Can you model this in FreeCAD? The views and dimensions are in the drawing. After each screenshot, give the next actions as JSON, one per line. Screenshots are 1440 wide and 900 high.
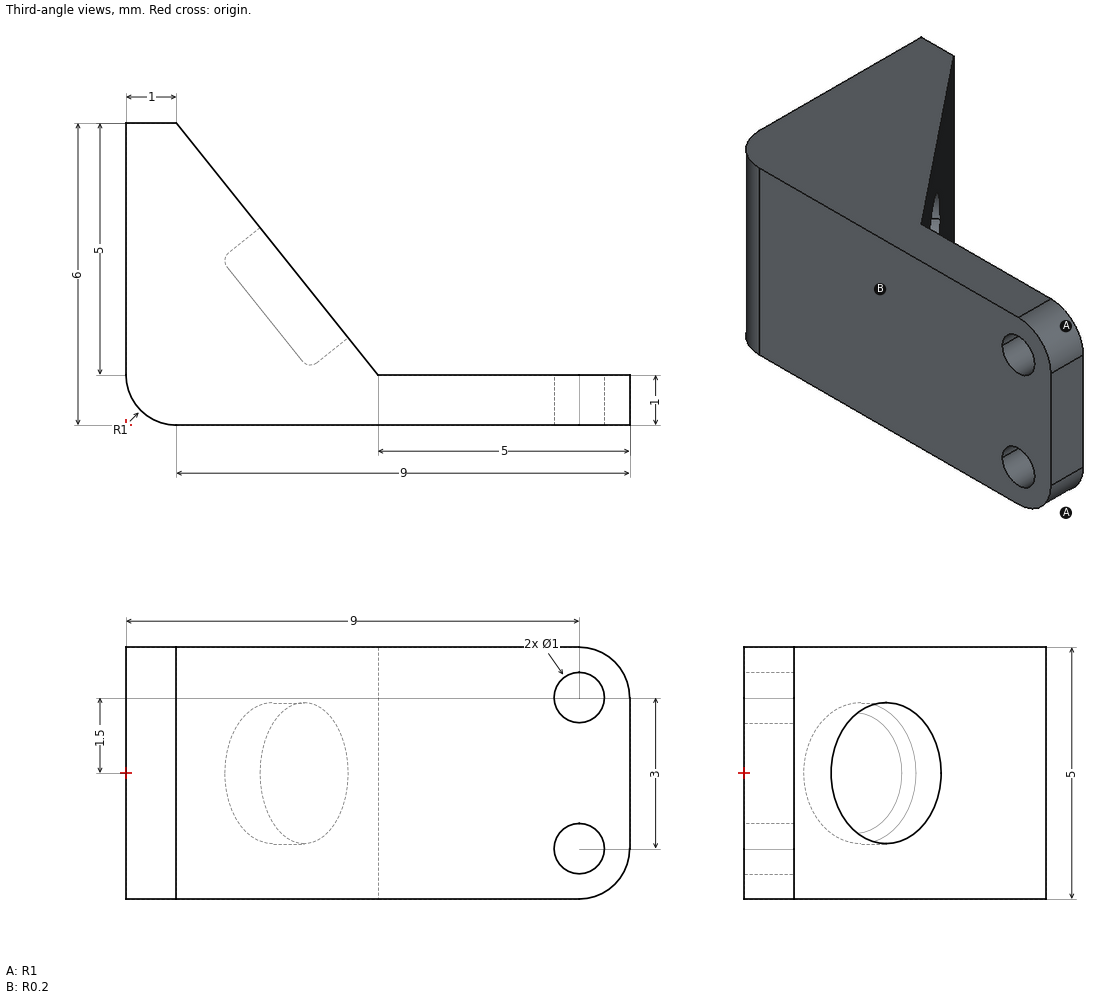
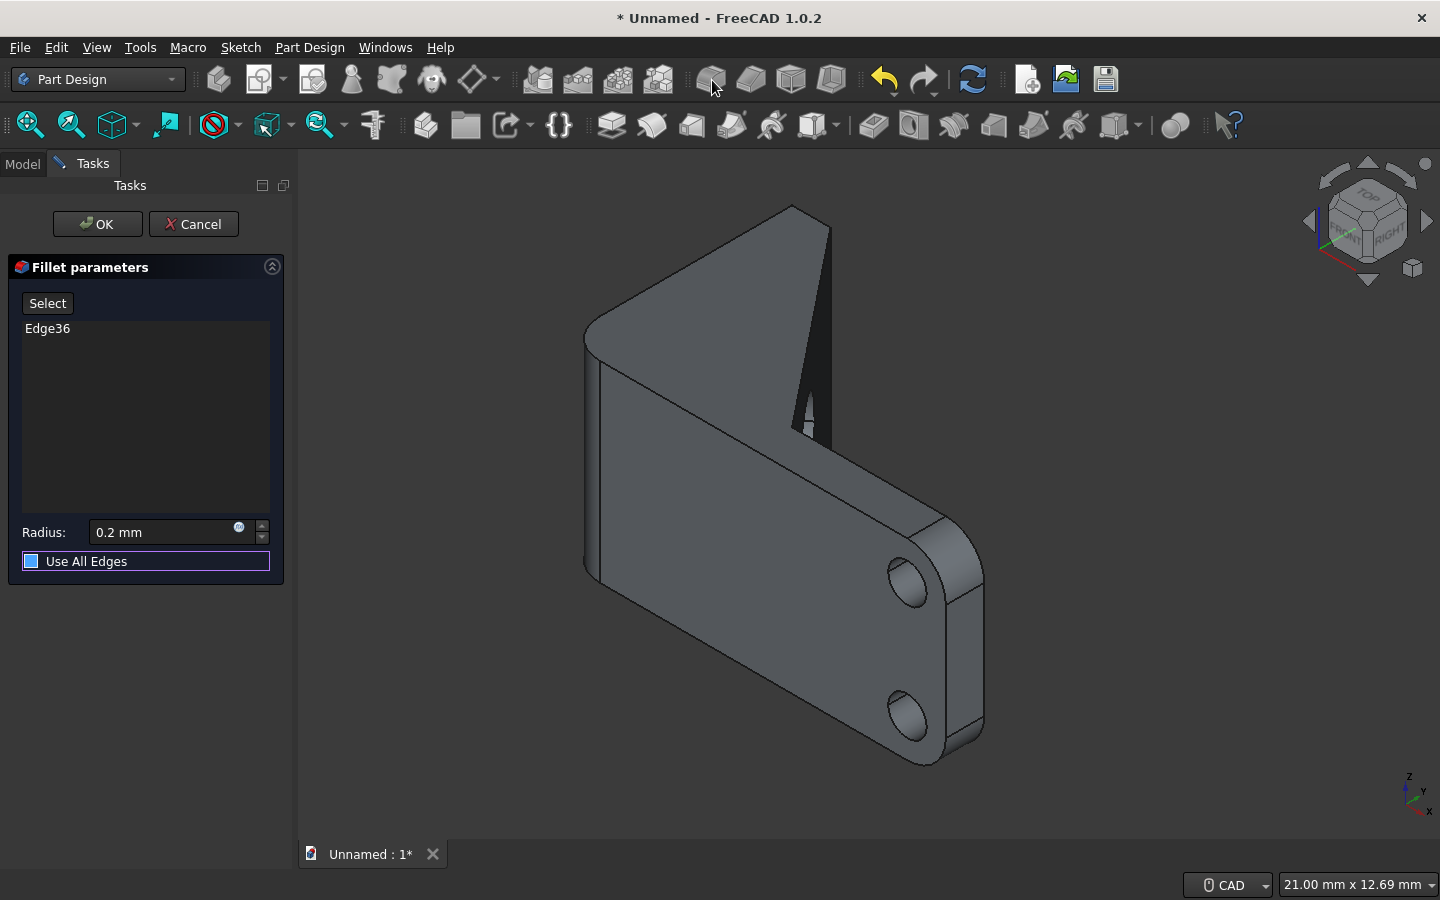
{"action": "left_click", "coordinate": [98, 224]}